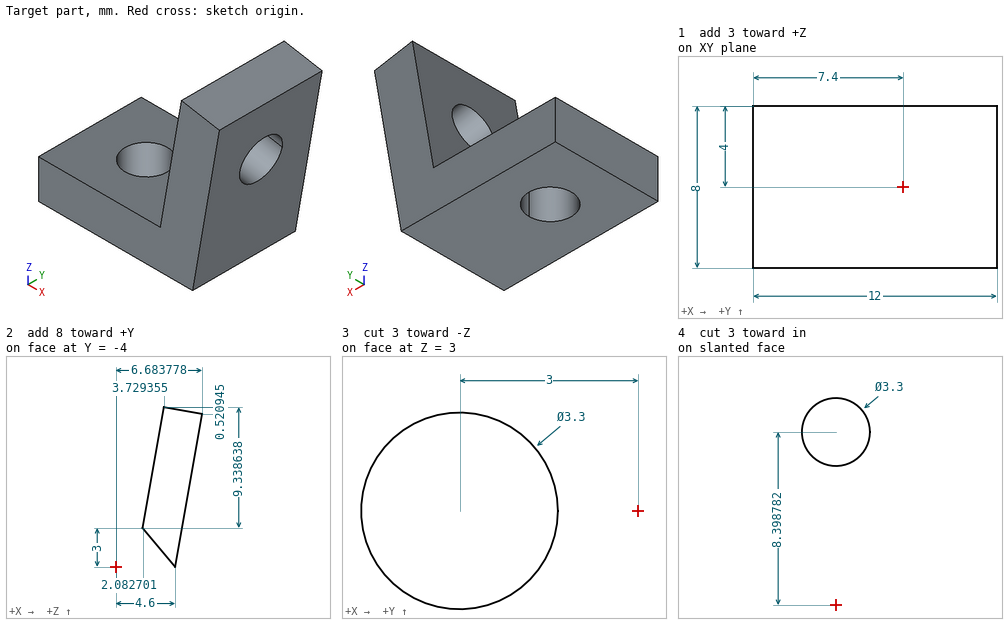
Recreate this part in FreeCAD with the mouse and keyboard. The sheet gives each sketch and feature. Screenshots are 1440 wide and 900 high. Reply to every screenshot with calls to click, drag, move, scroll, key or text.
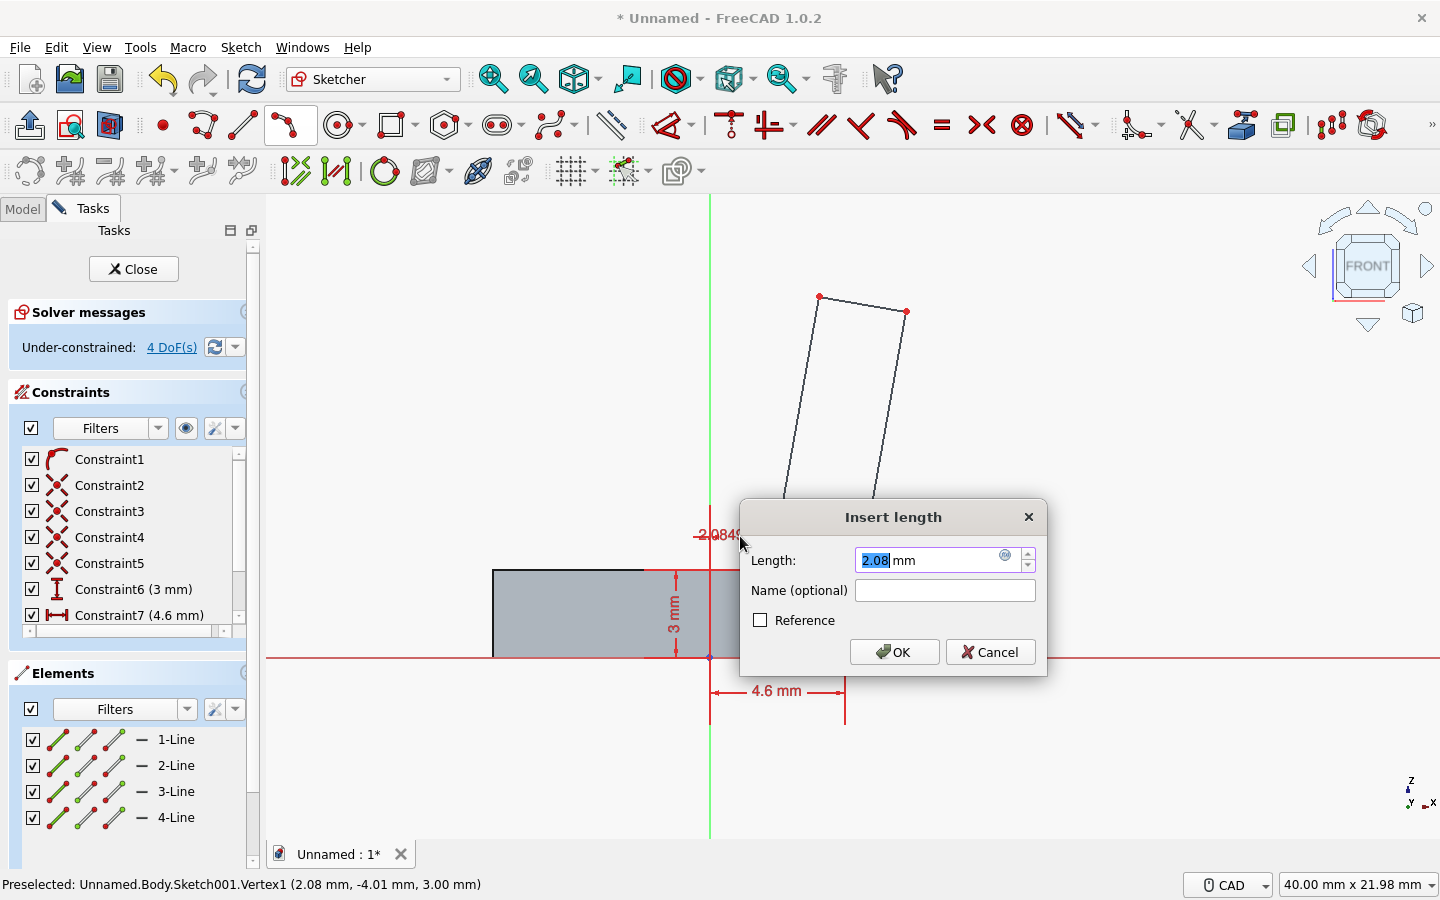
text(2.082701)
key(Return)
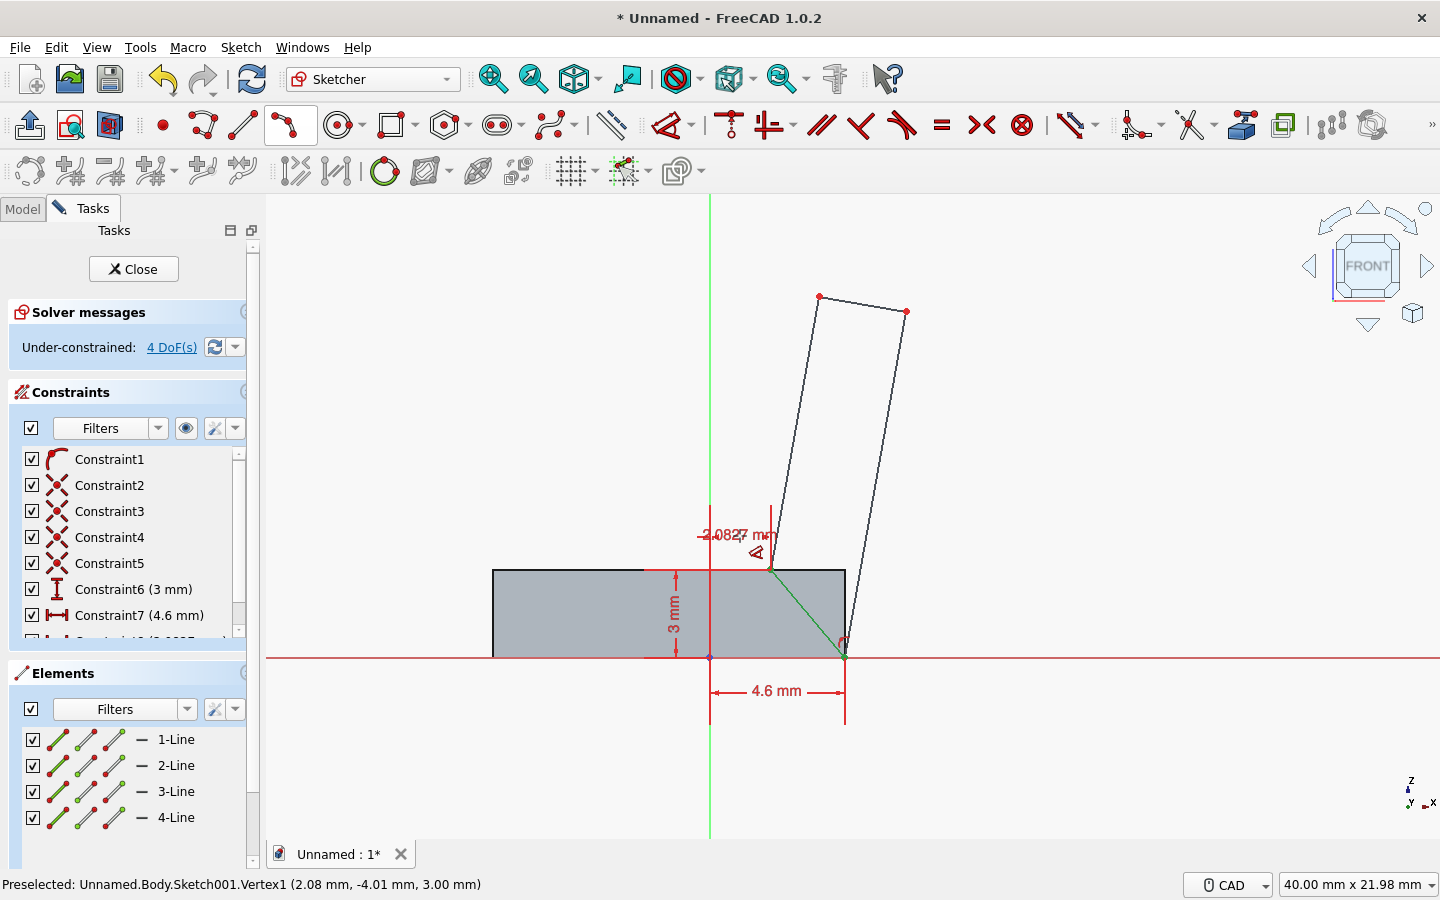
click(906, 312)
click(853, 692)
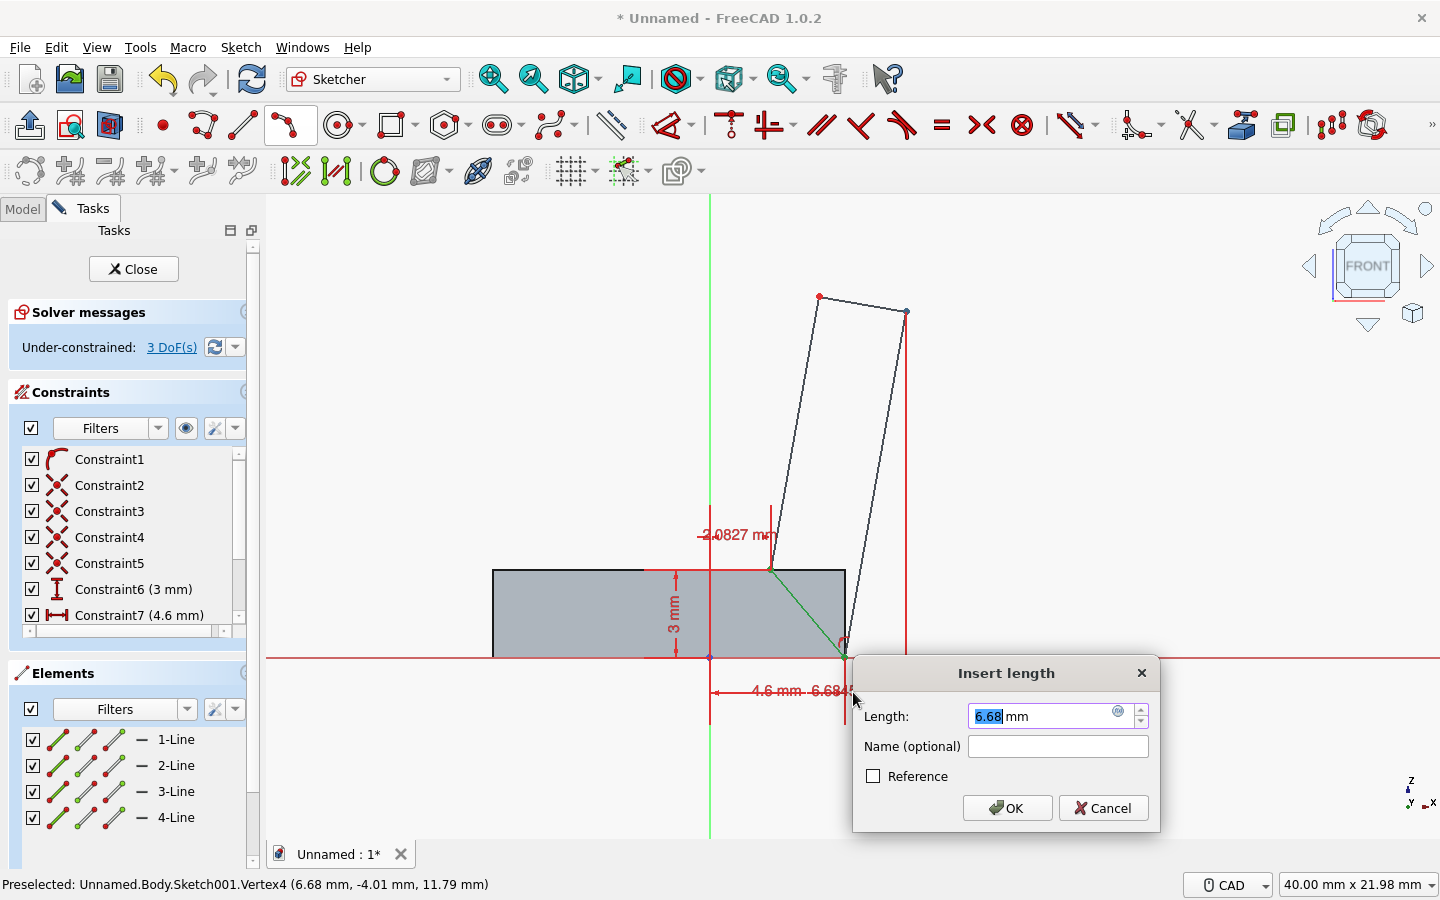
text(6.683778)
key(Return)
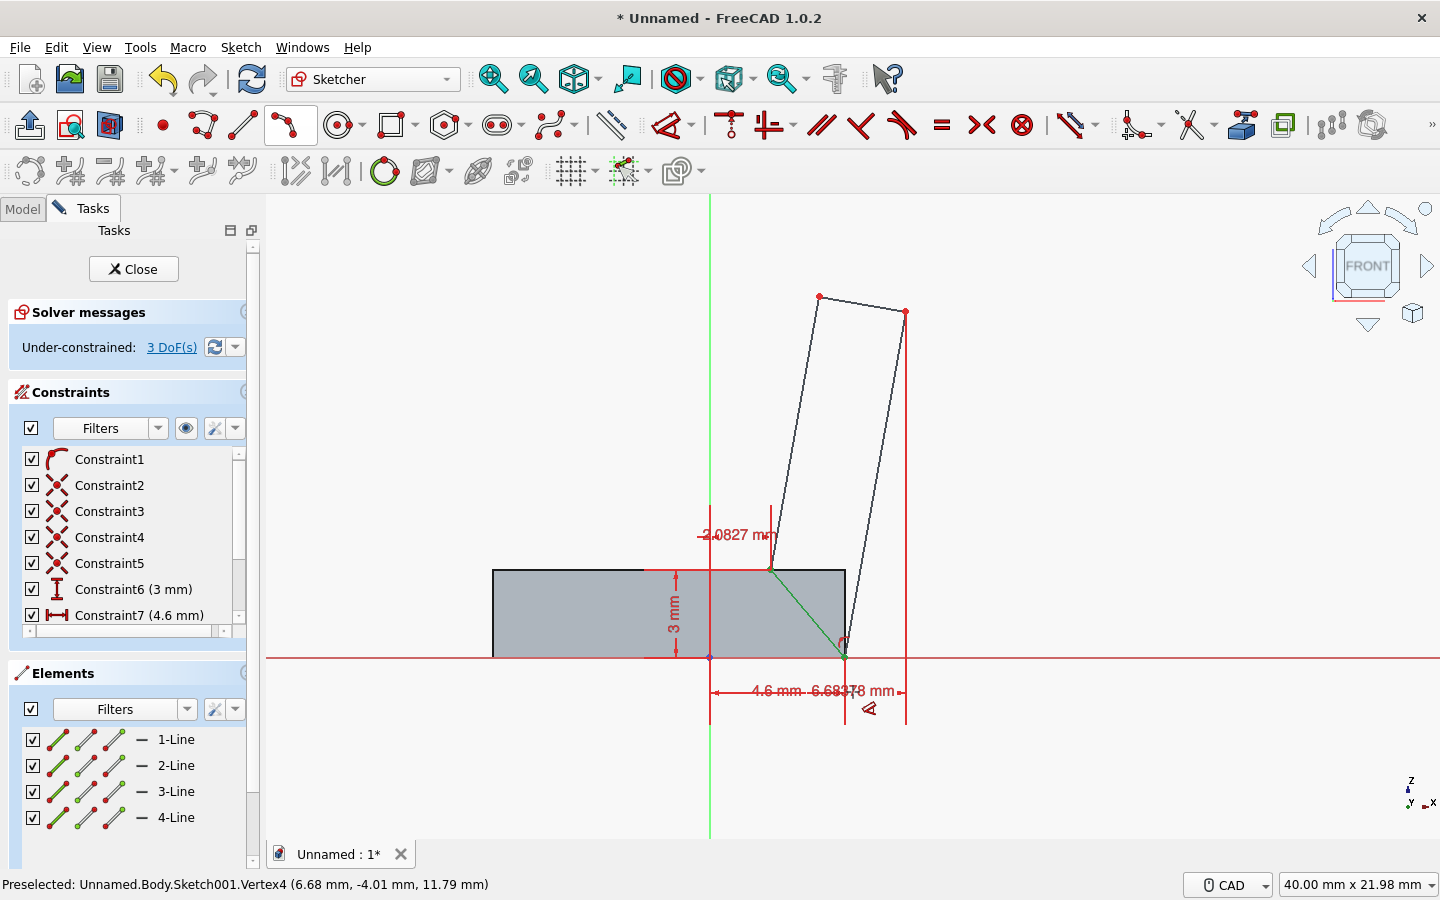
click(819, 297)
click(764, 263)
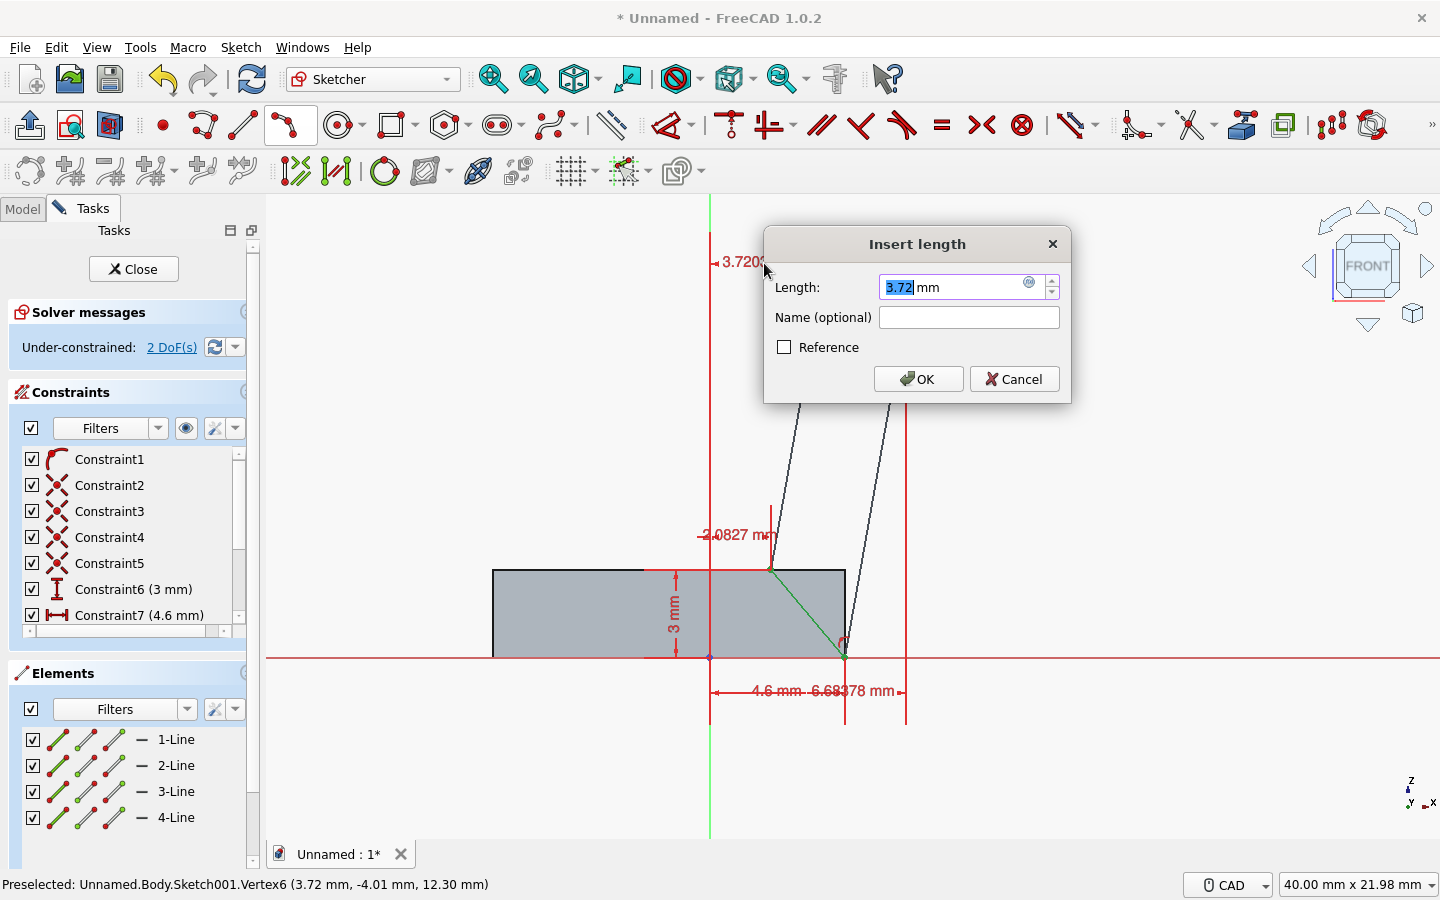
text(3.729355)
key(Return)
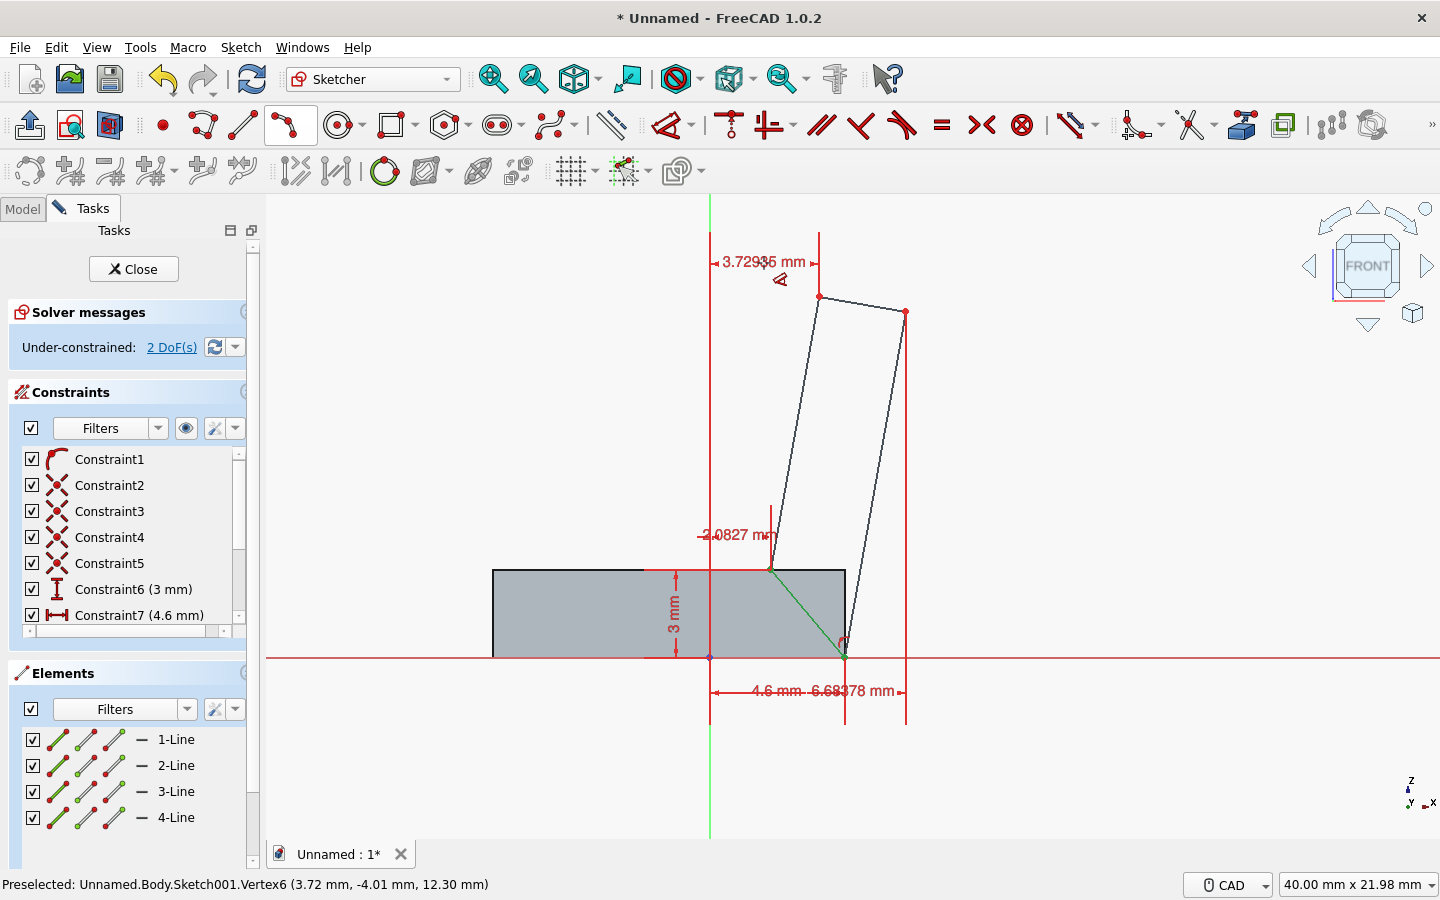
scroll(880, 307, up, 5)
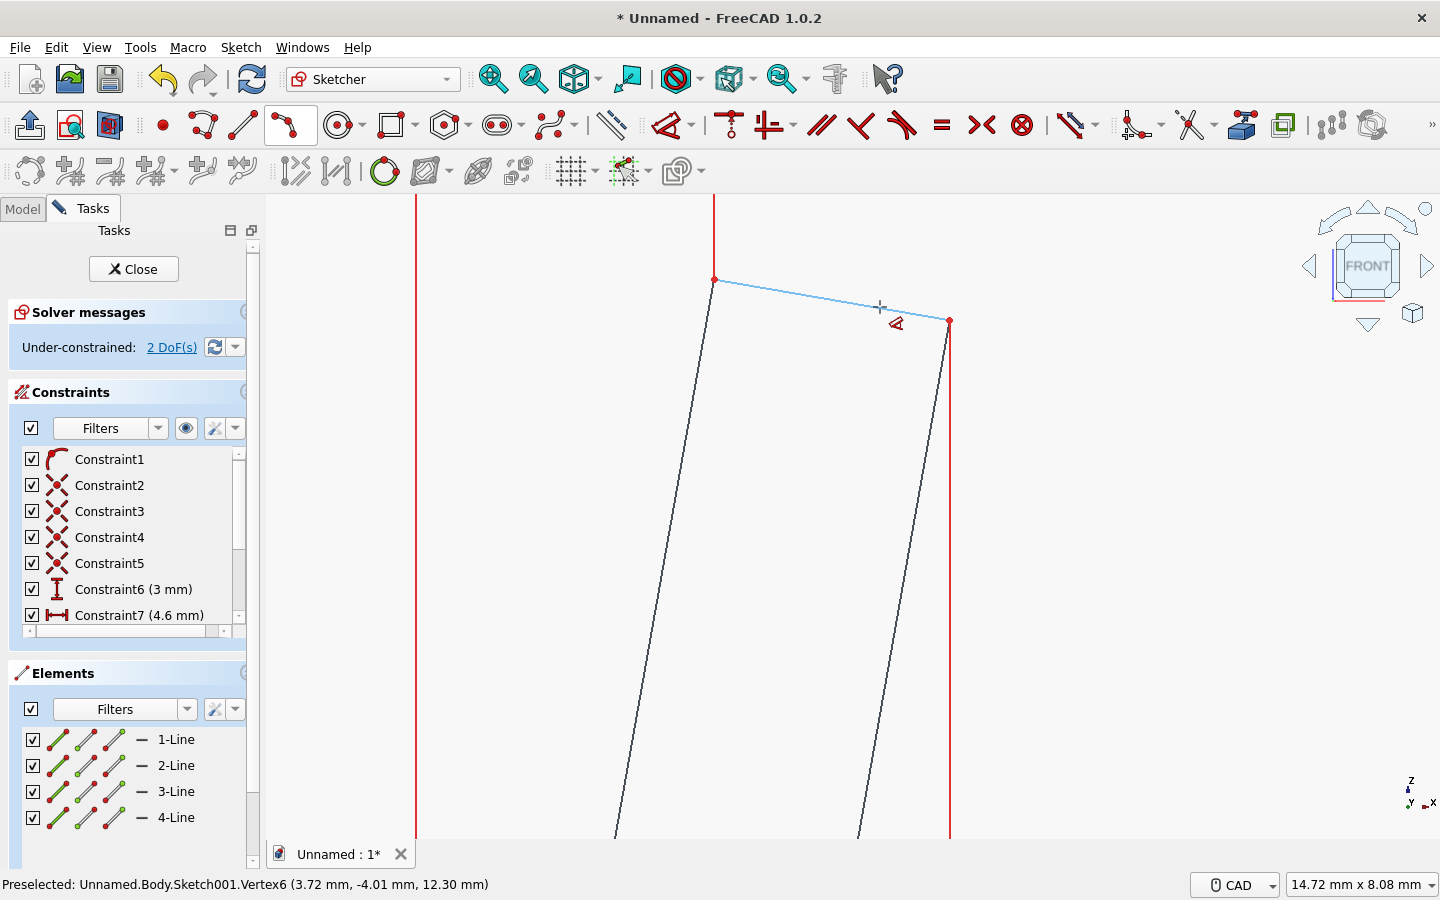
click(879, 308)
click(984, 300)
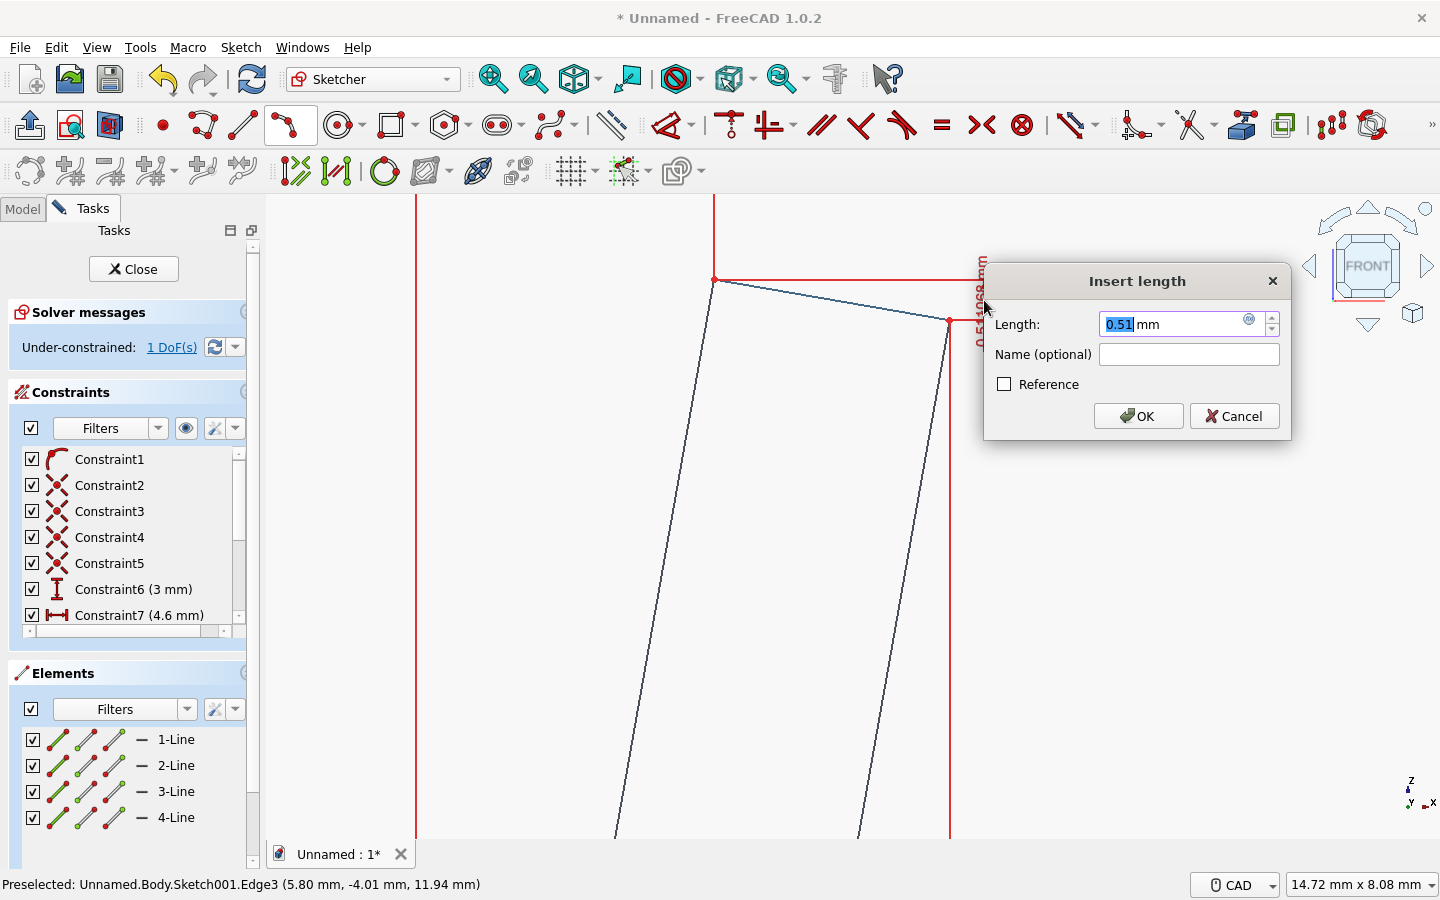
text(0.520945)
key(Return)